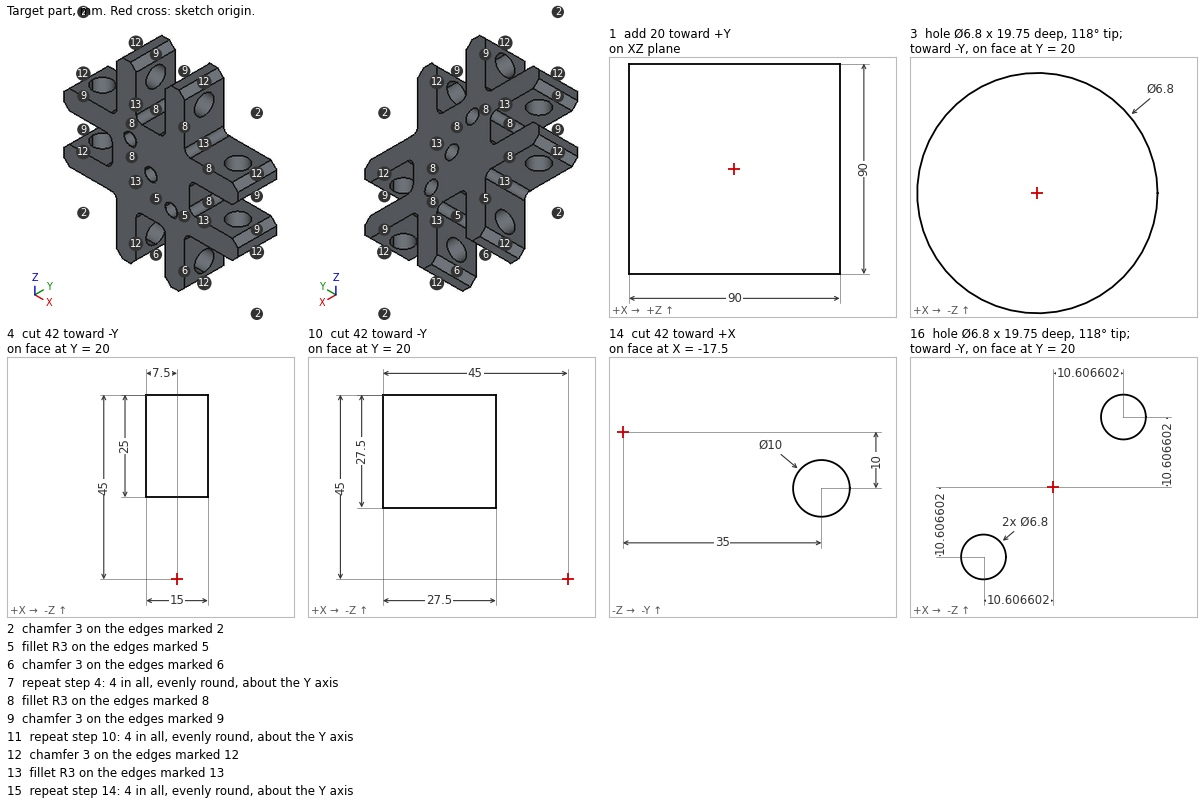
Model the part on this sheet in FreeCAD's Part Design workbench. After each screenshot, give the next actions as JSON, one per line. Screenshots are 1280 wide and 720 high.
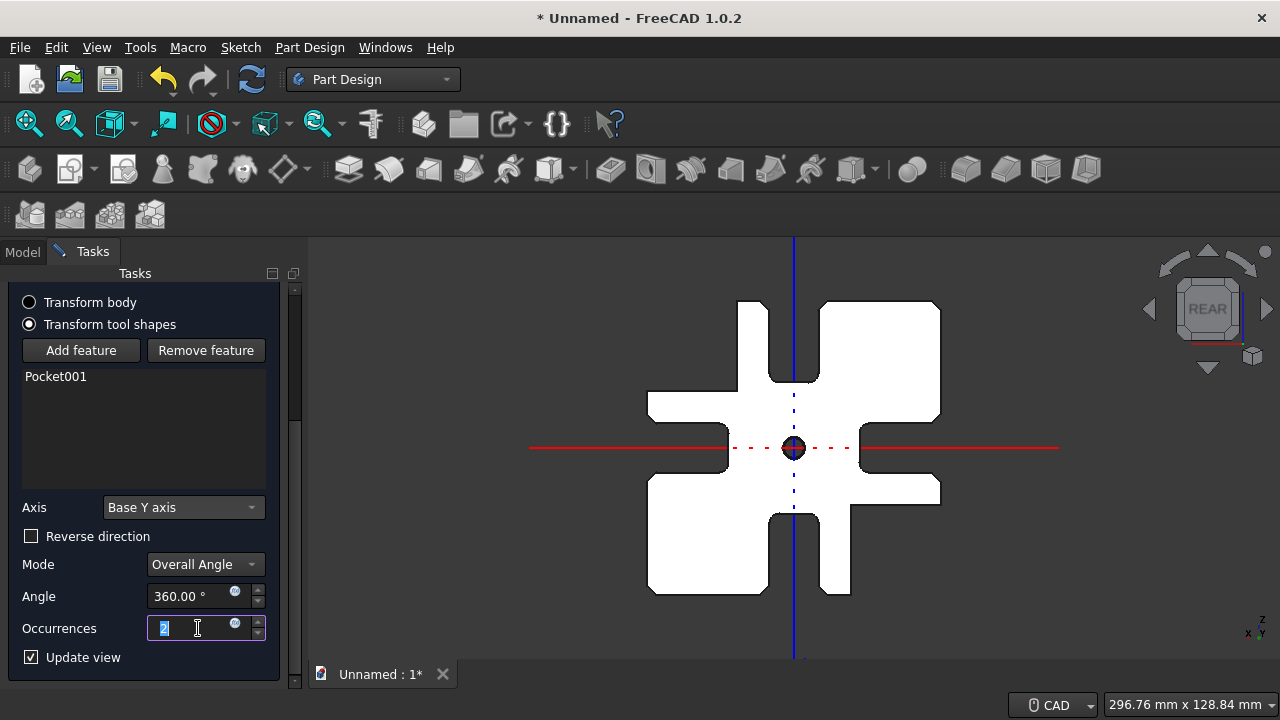
{"action": "type", "text": "4"}
{"action": "key", "text": "Tab"}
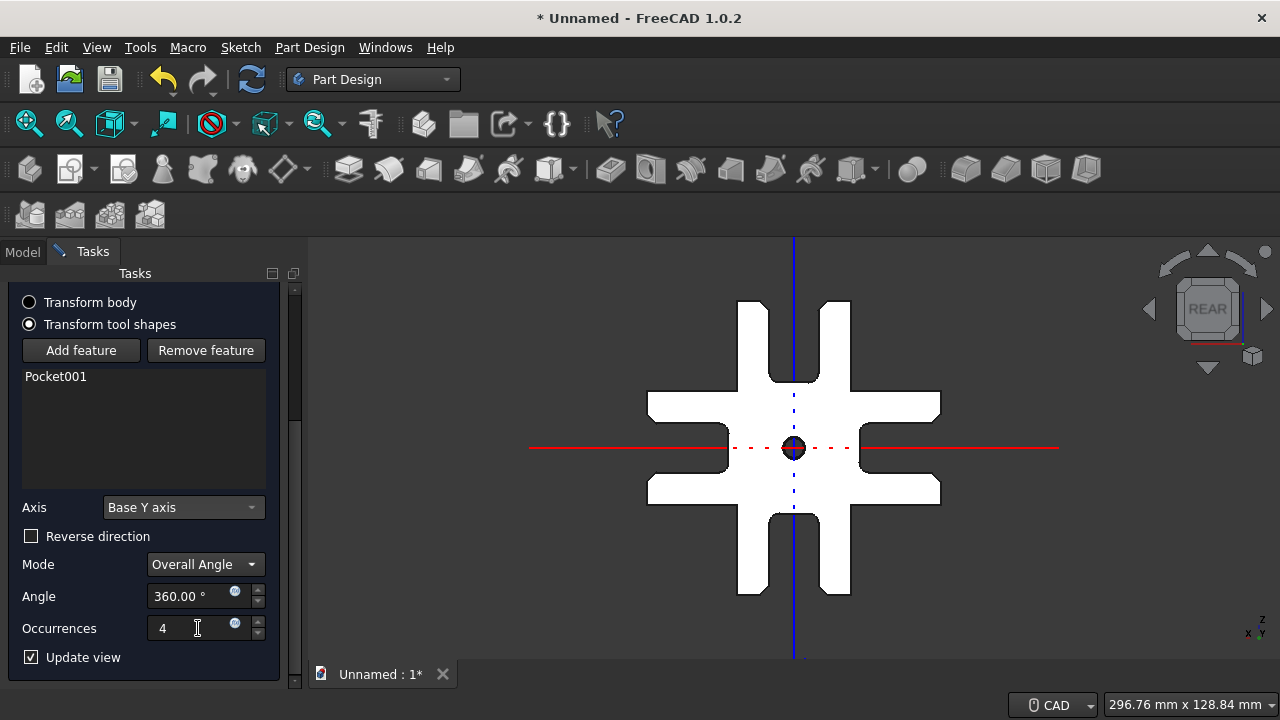
{"action": "scroll", "coordinate": [295, 486], "scroll_direction": "up", "scroll_amount": 5}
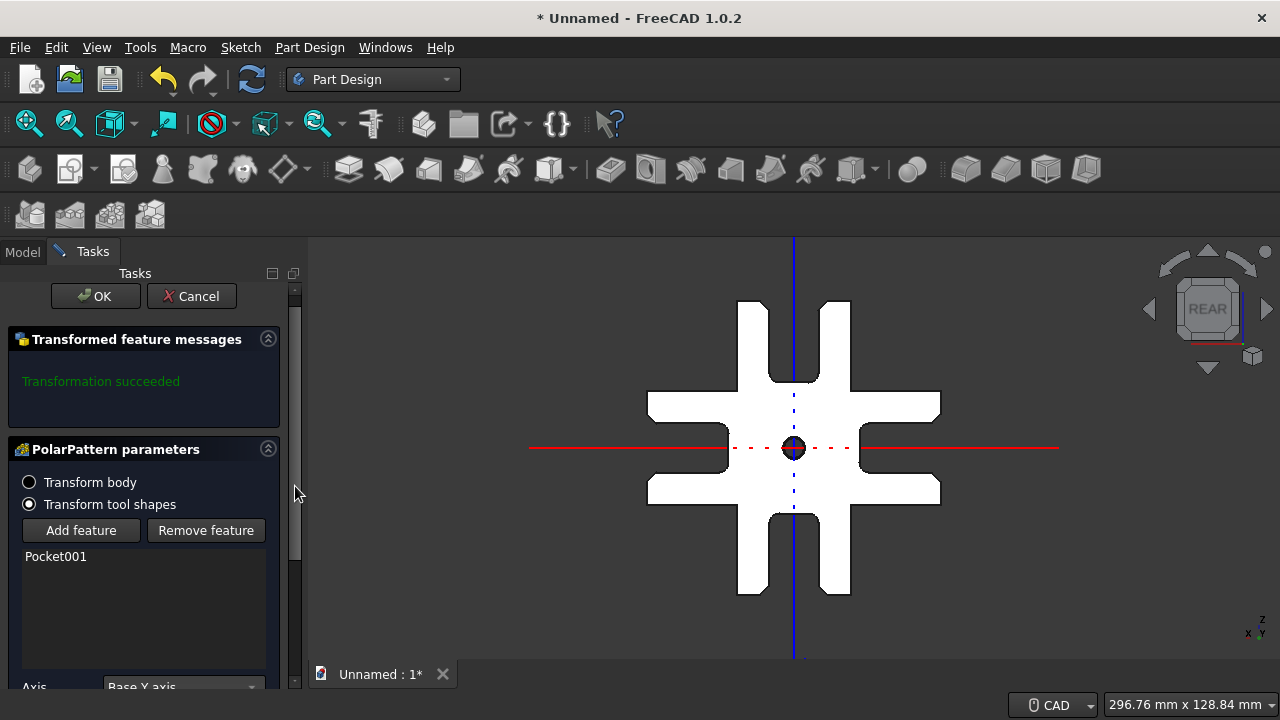
{"action": "left_click", "coordinate": [96, 312]}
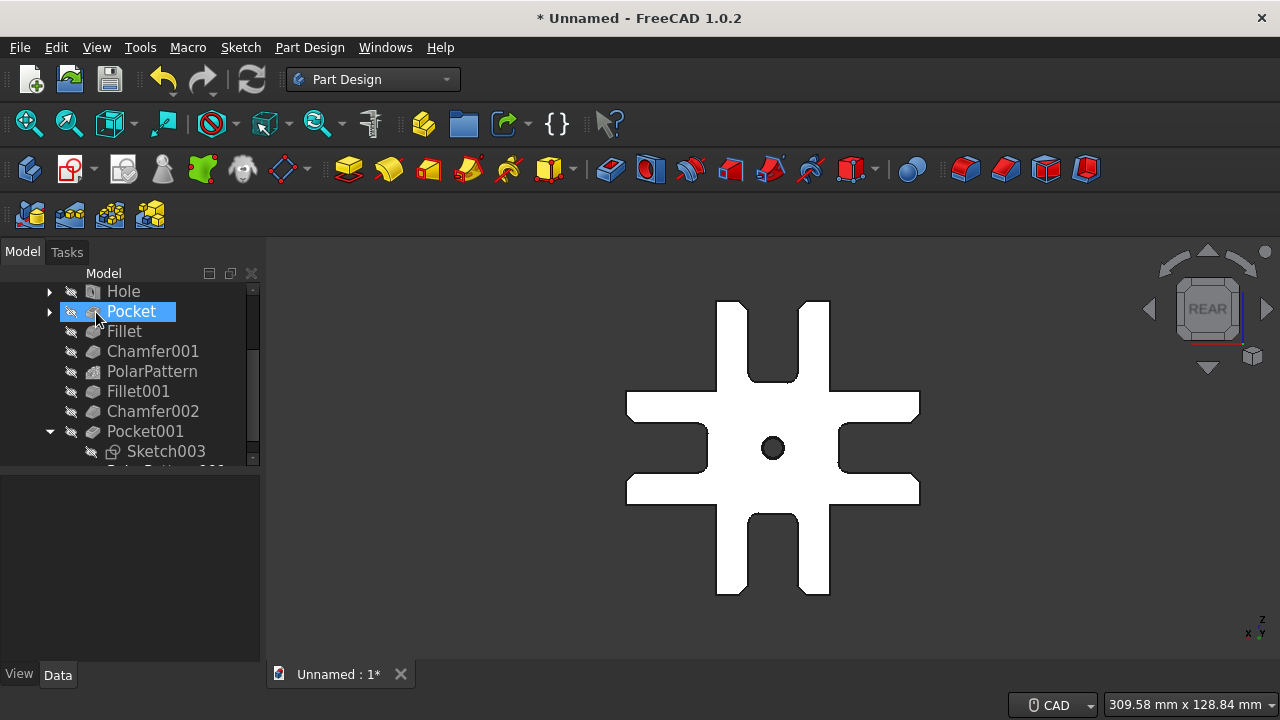
{"action": "key", "text": "0"}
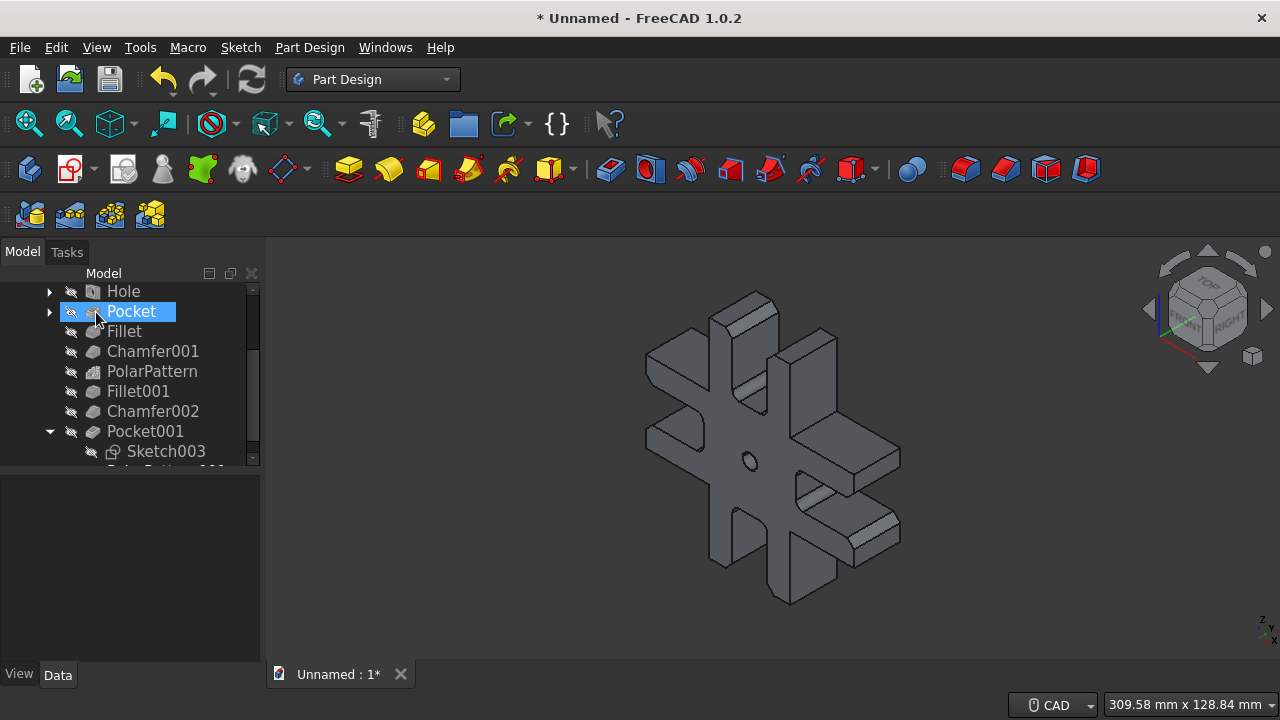
{"action": "left_click", "coordinate": [814, 350]}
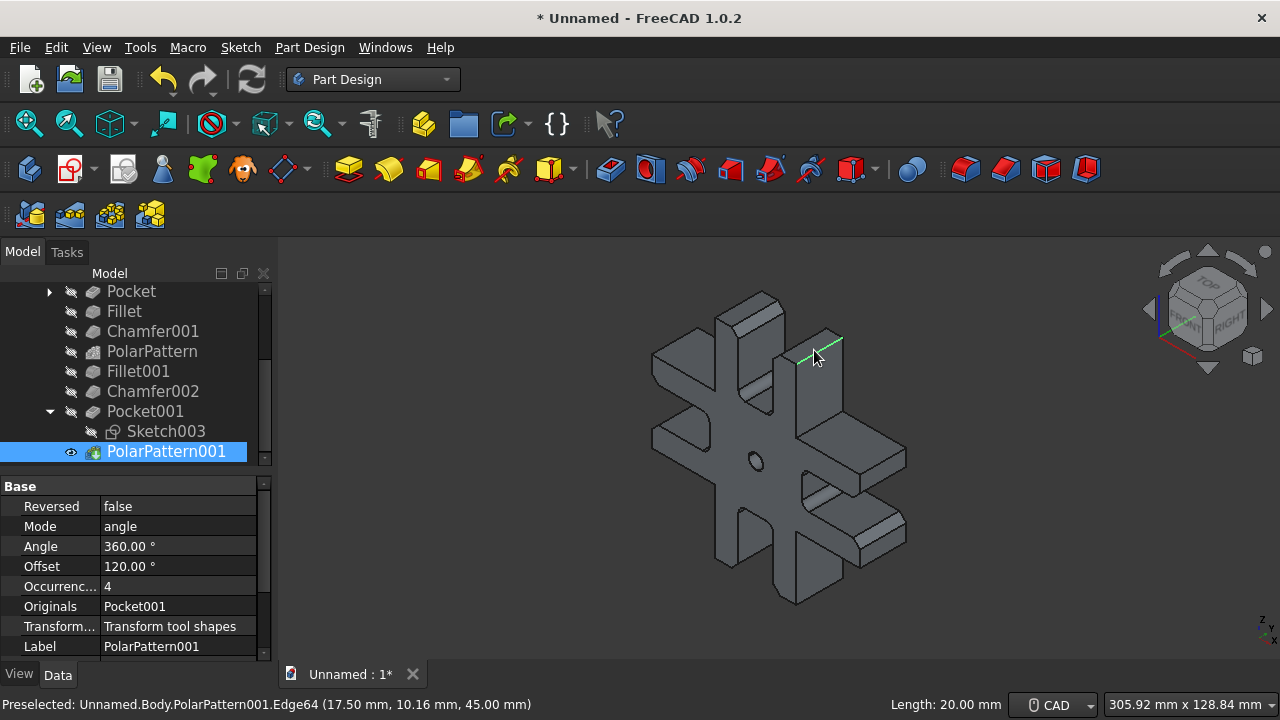
{"action": "left_click", "coordinate": [883, 460], "text": "ctrl"}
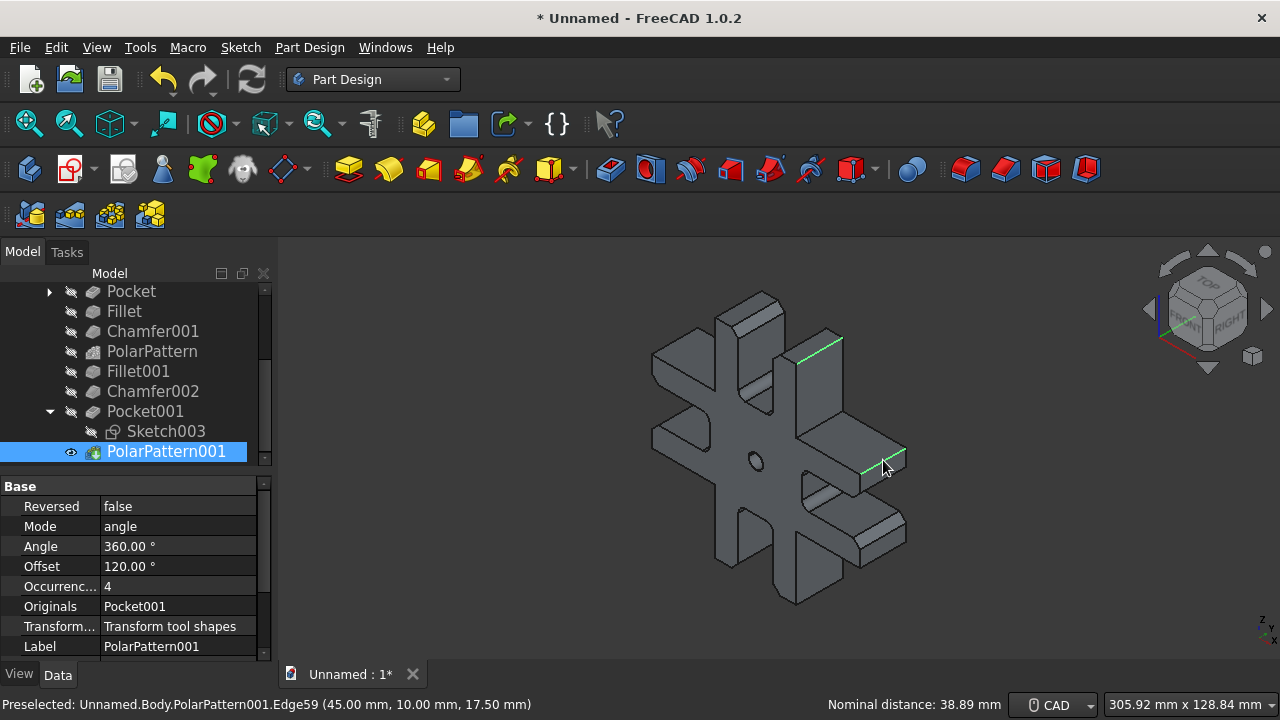
{"action": "key", "text": "2"}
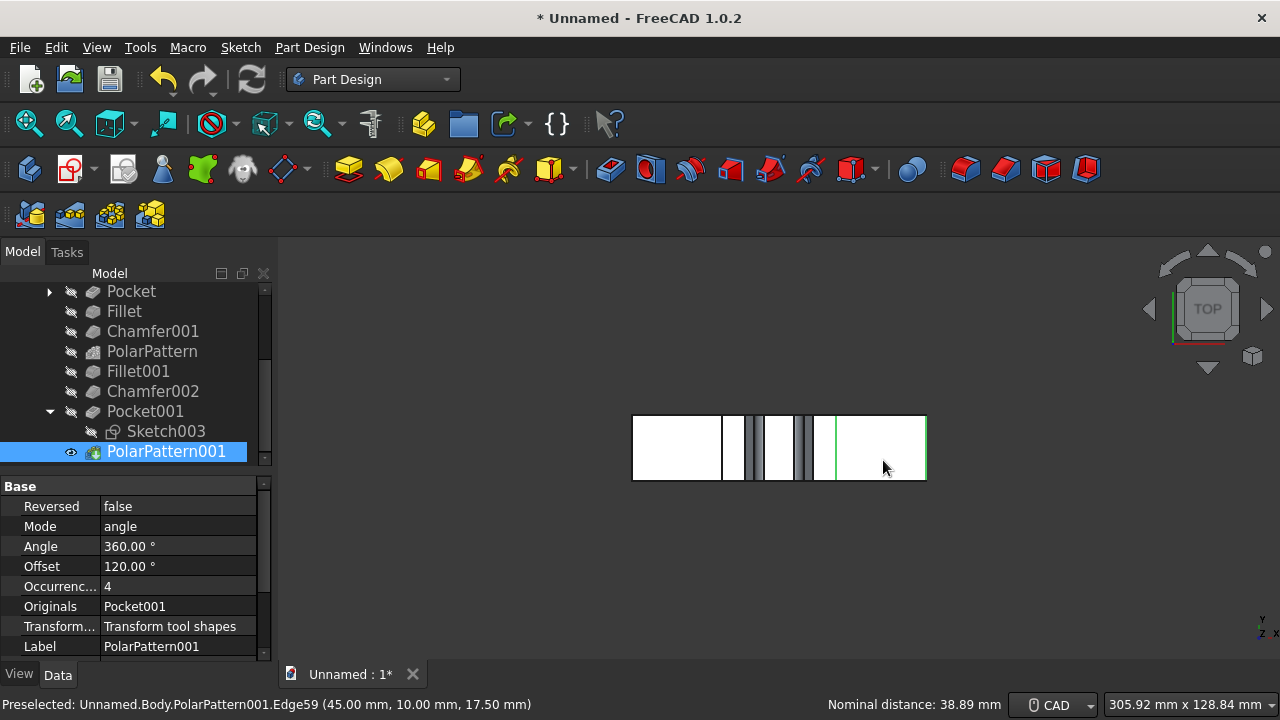
{"action": "left_click", "coordinate": [30, 124]}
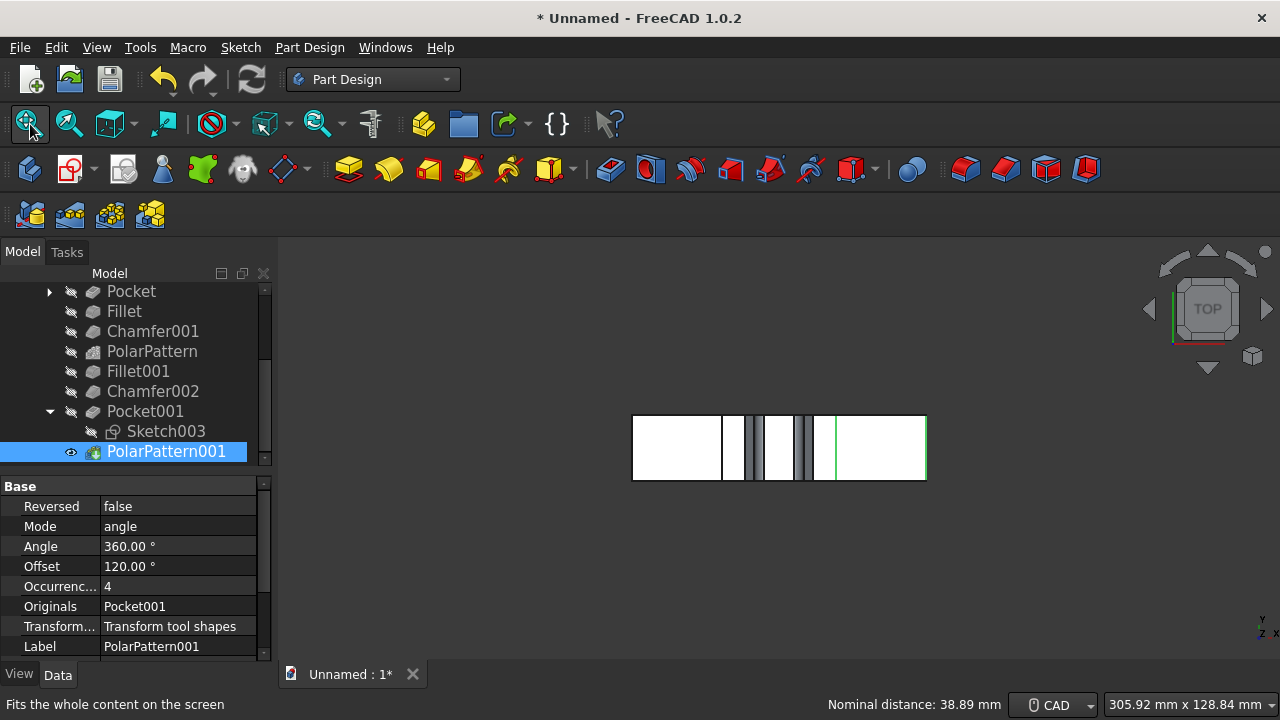
{"action": "left_click", "coordinate": [632, 447], "text": "ctrl"}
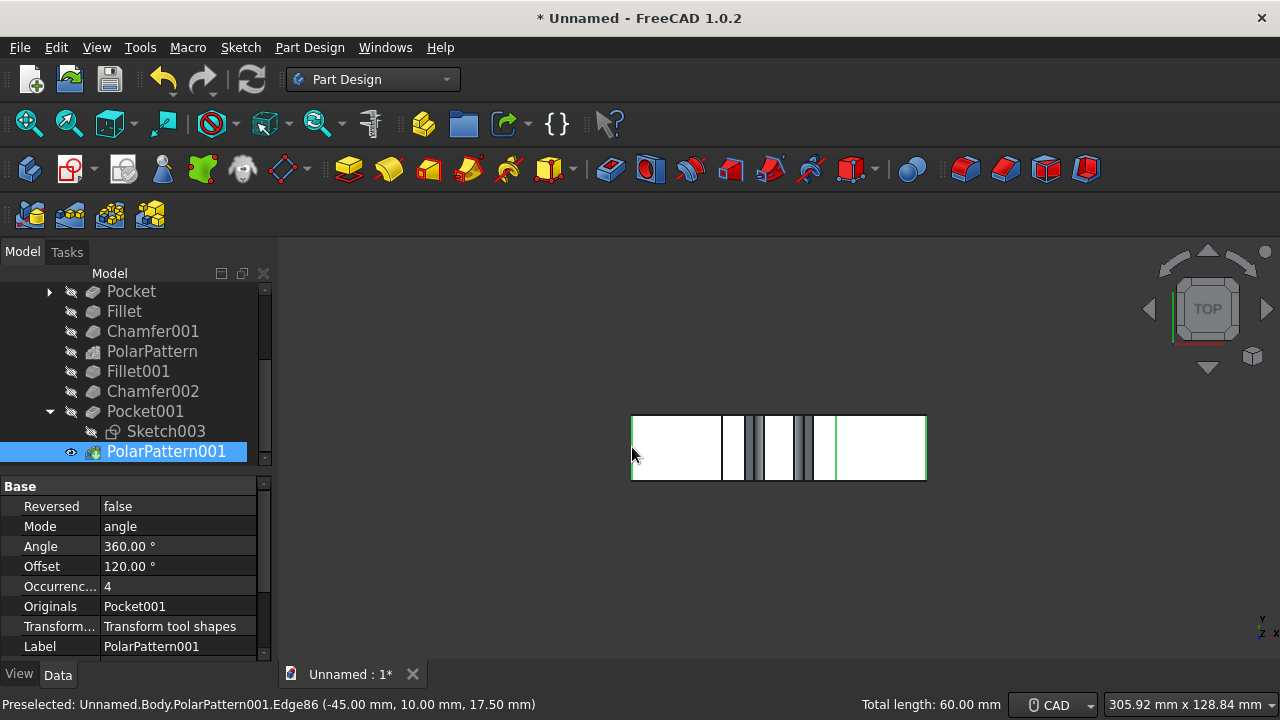
{"action": "left_click", "coordinate": [722, 447], "text": "ctrl"}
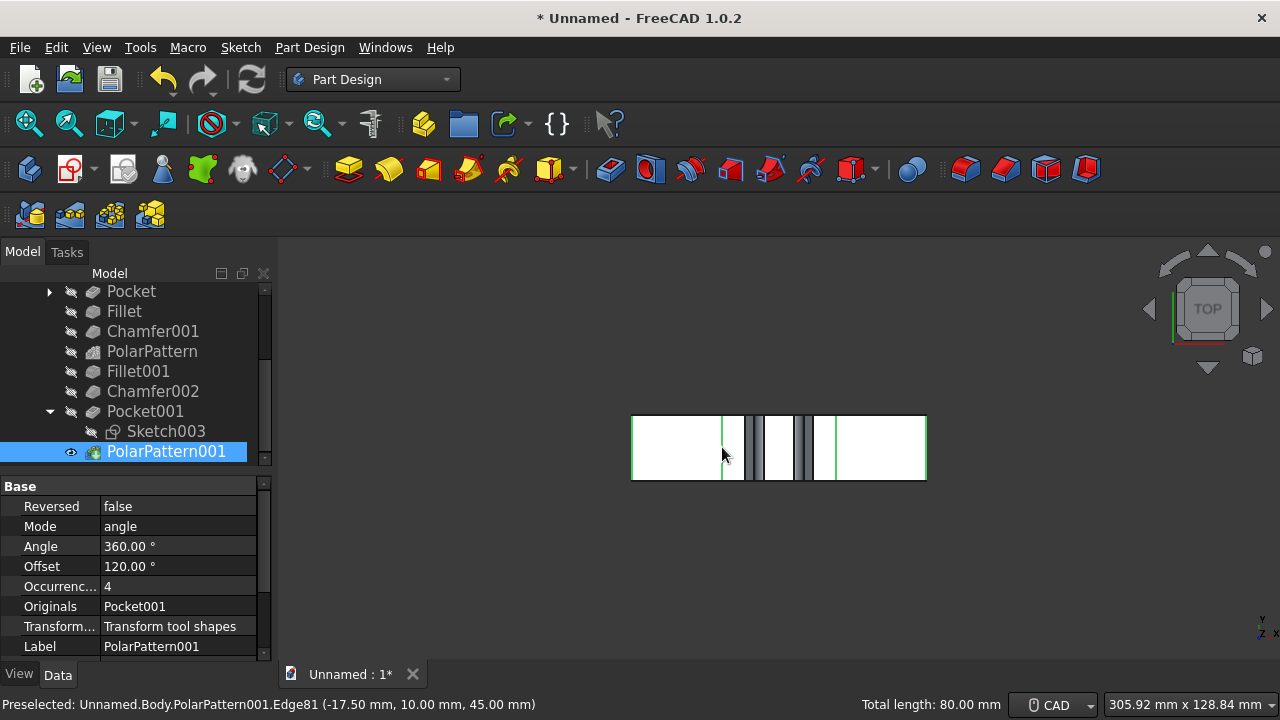
{"action": "key", "text": "1"}